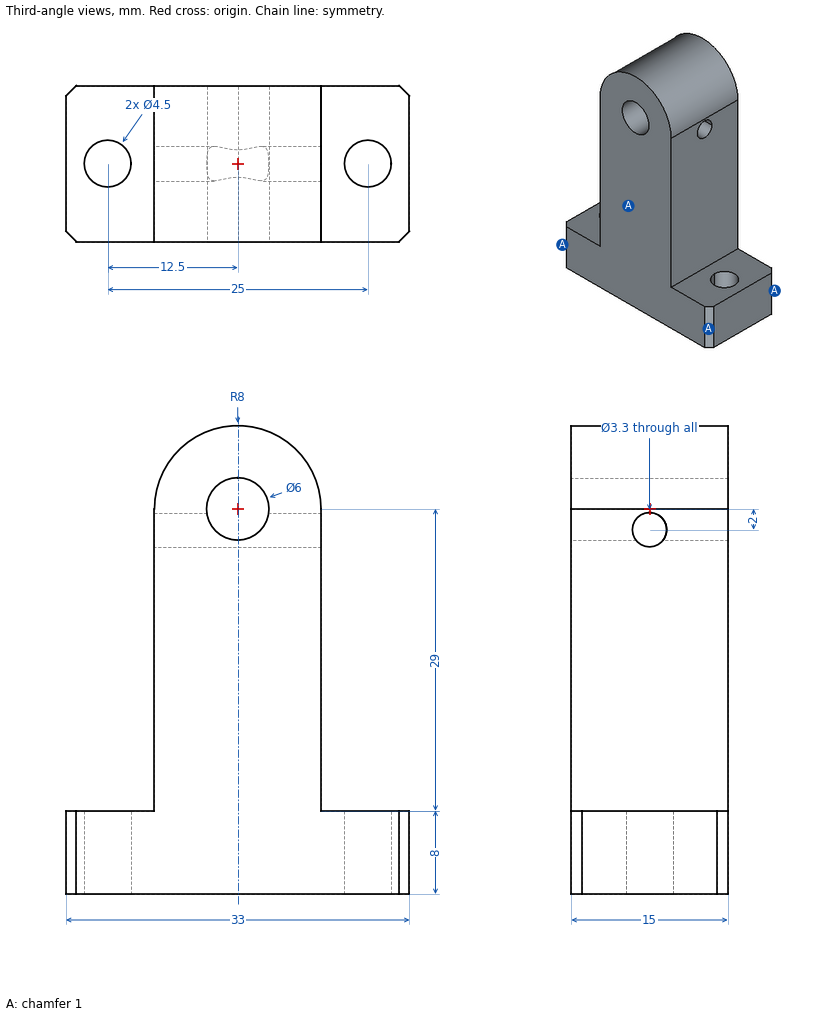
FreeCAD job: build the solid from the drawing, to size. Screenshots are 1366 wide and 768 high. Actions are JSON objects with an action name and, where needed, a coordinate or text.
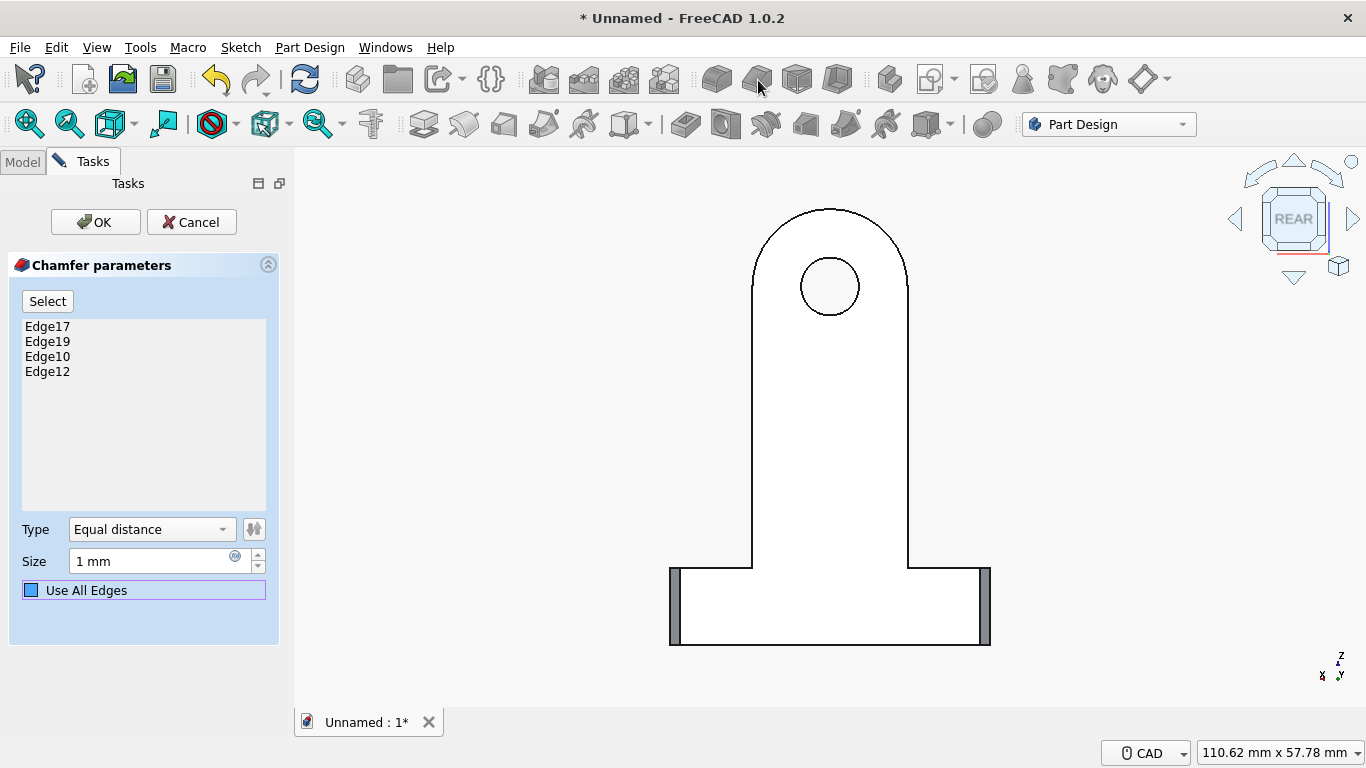
{"action": "left_click", "coordinate": [96, 222]}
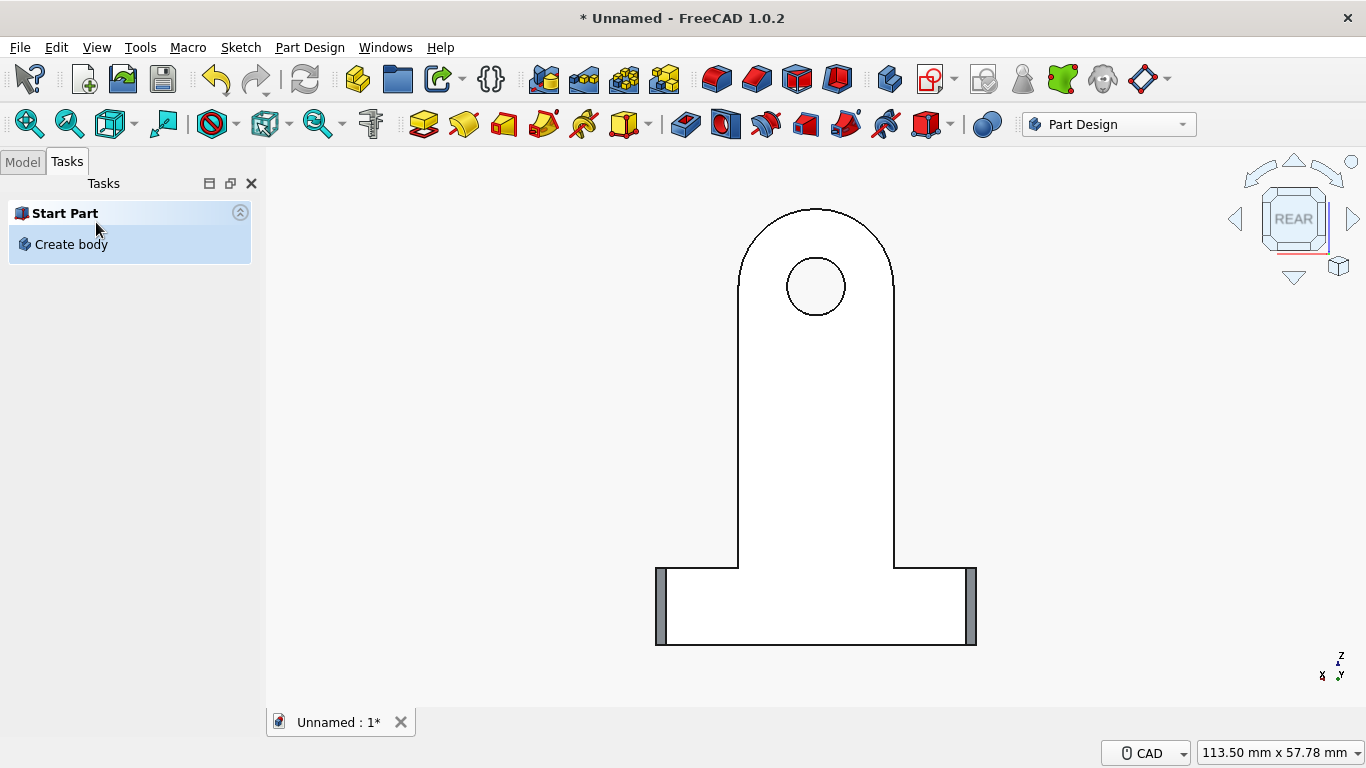
{"action": "key", "text": "0"}